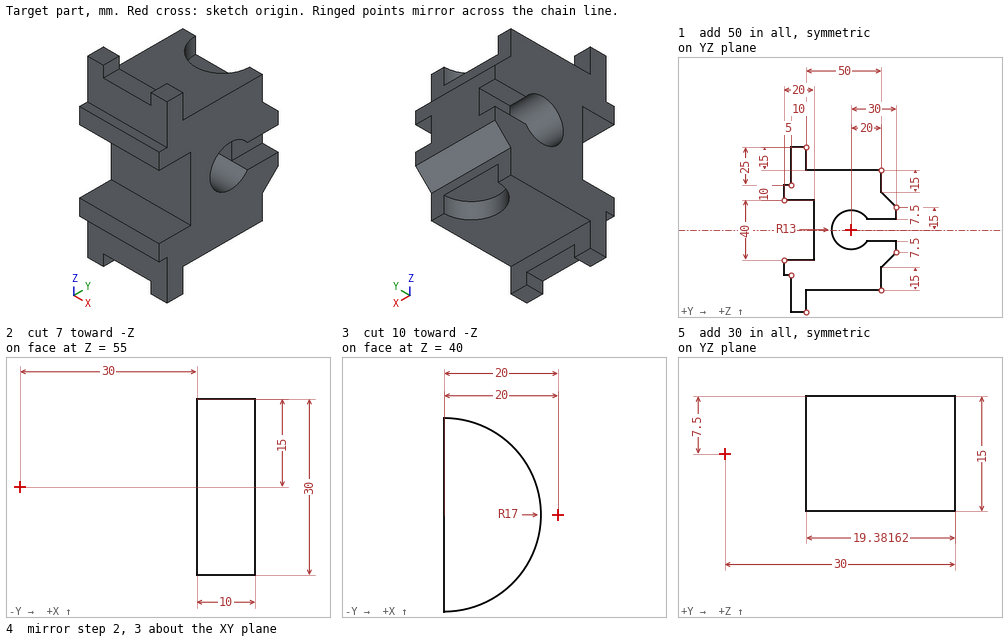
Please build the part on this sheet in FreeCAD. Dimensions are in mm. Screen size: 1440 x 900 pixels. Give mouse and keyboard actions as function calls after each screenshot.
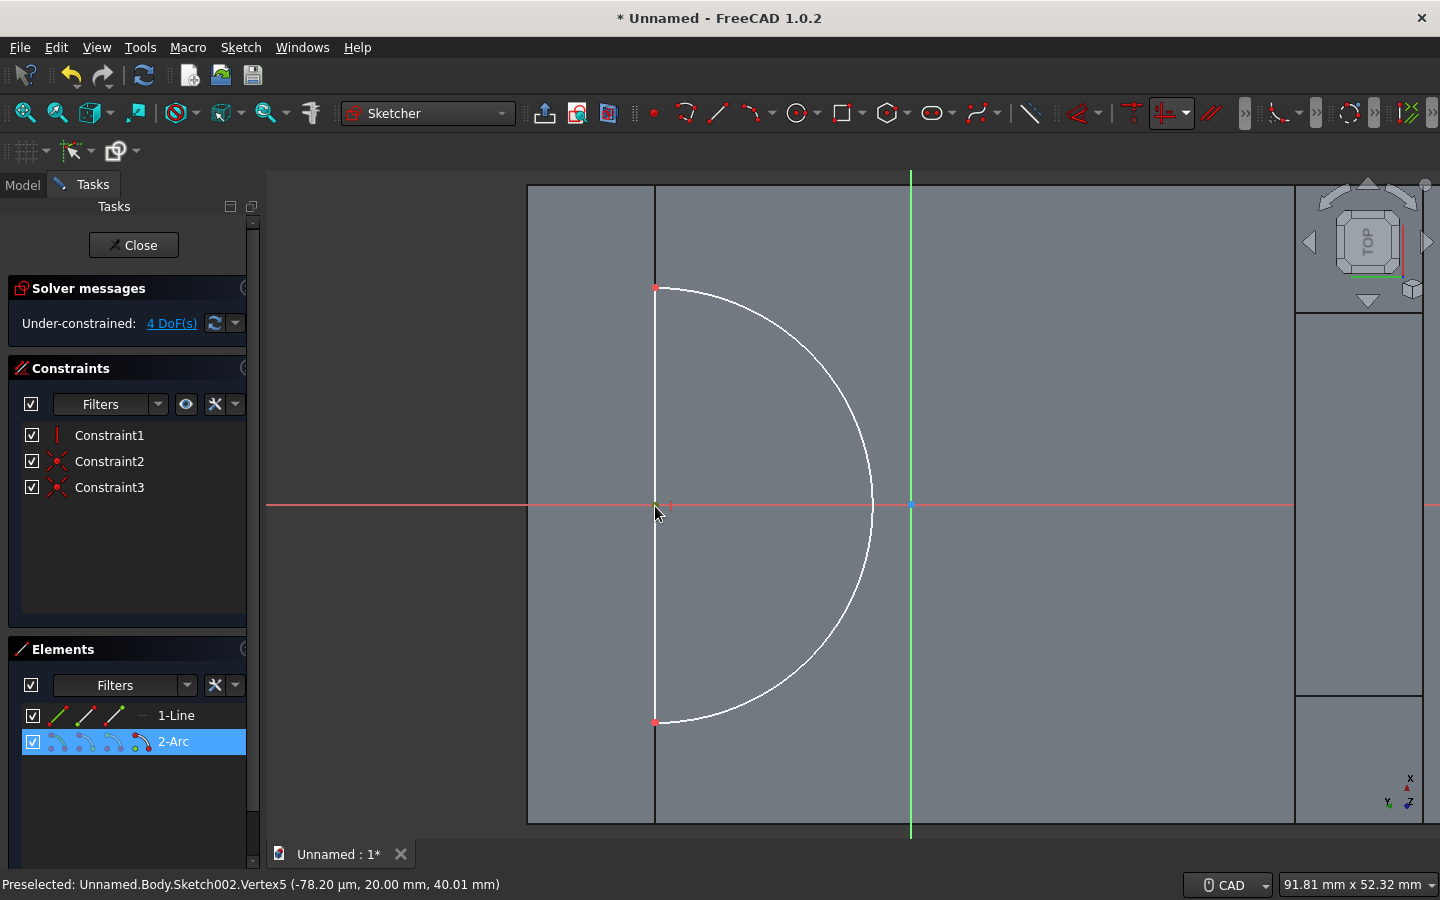
click(364, 504)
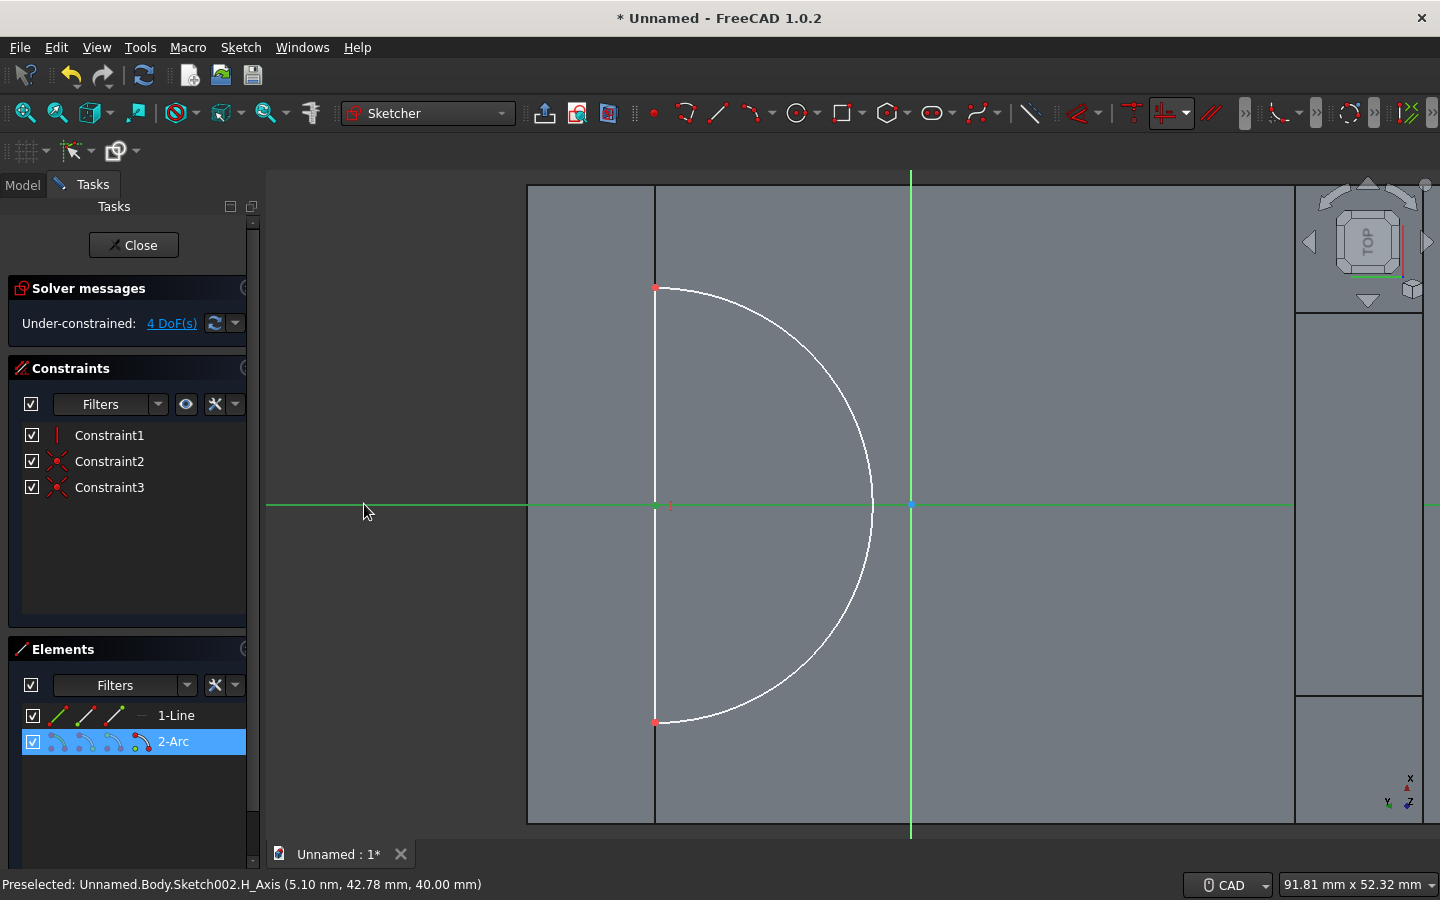
click(1132, 114)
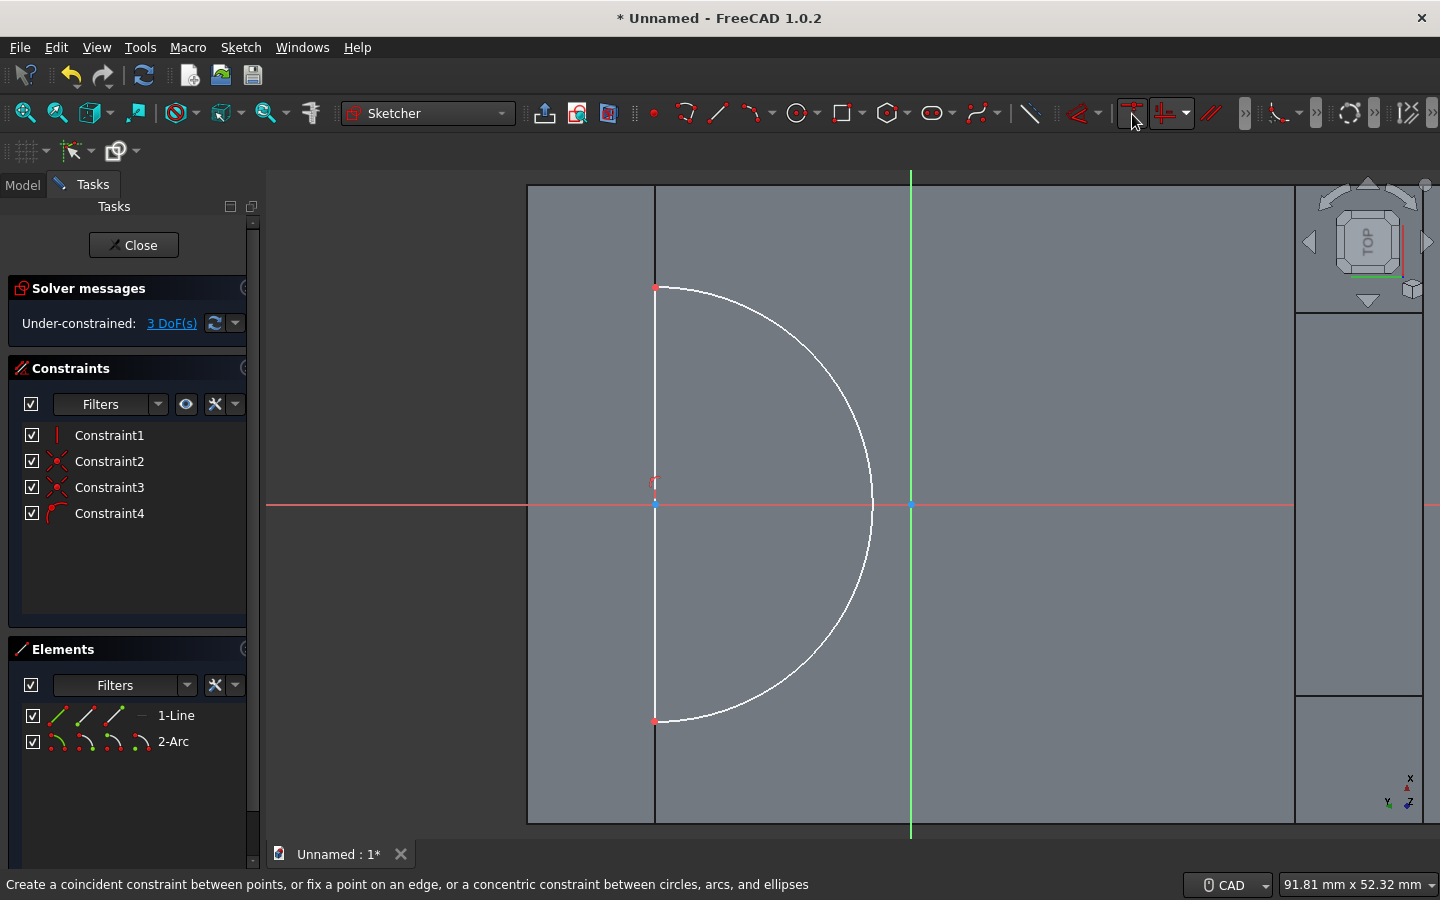
click(1078, 114)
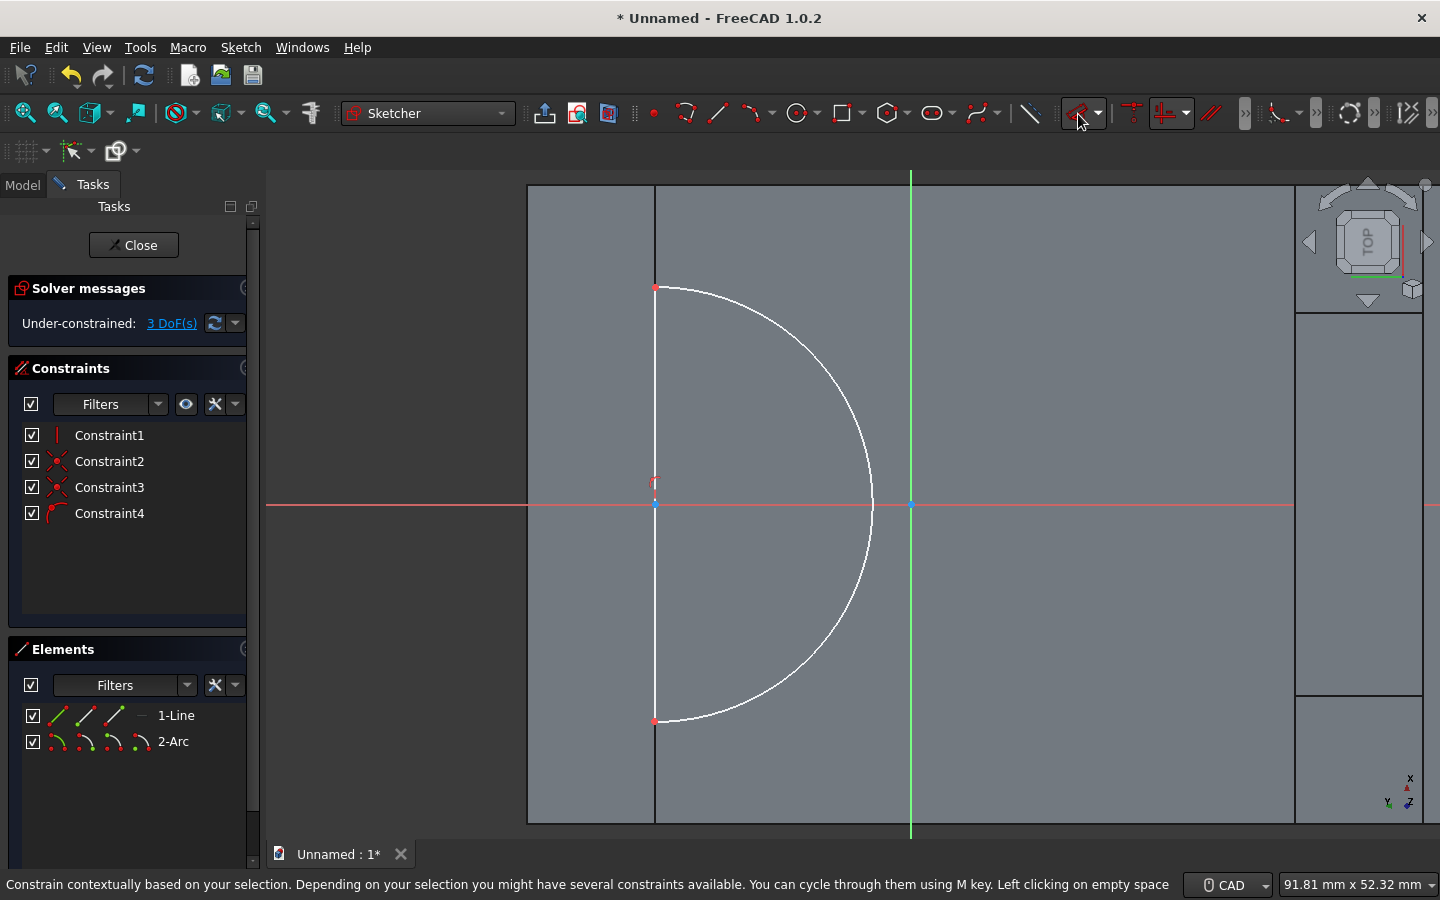
click(831, 632)
click(857, 651)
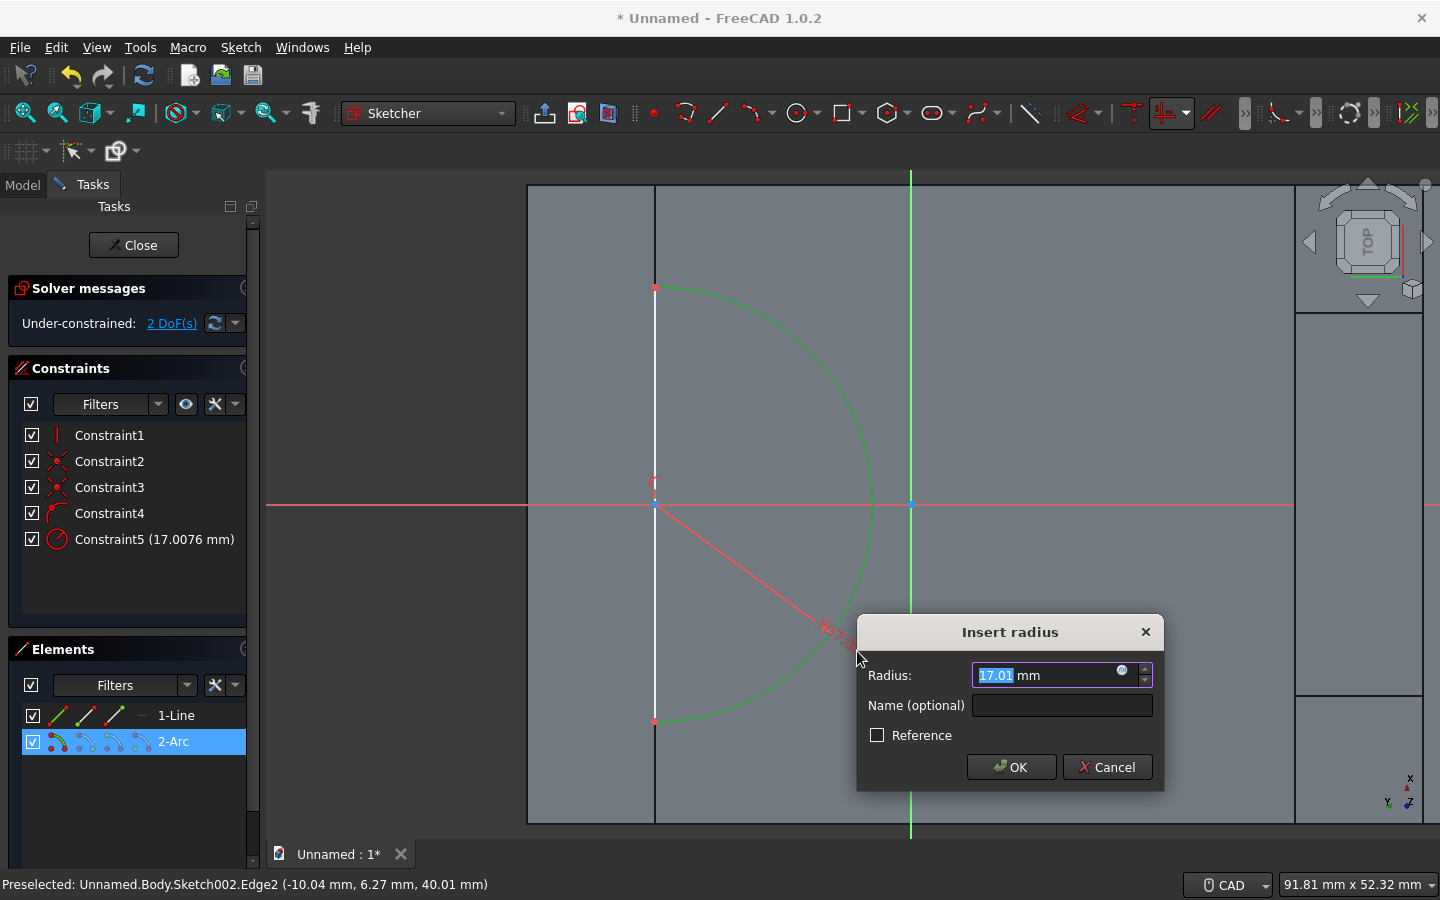
text(17)
key(Return)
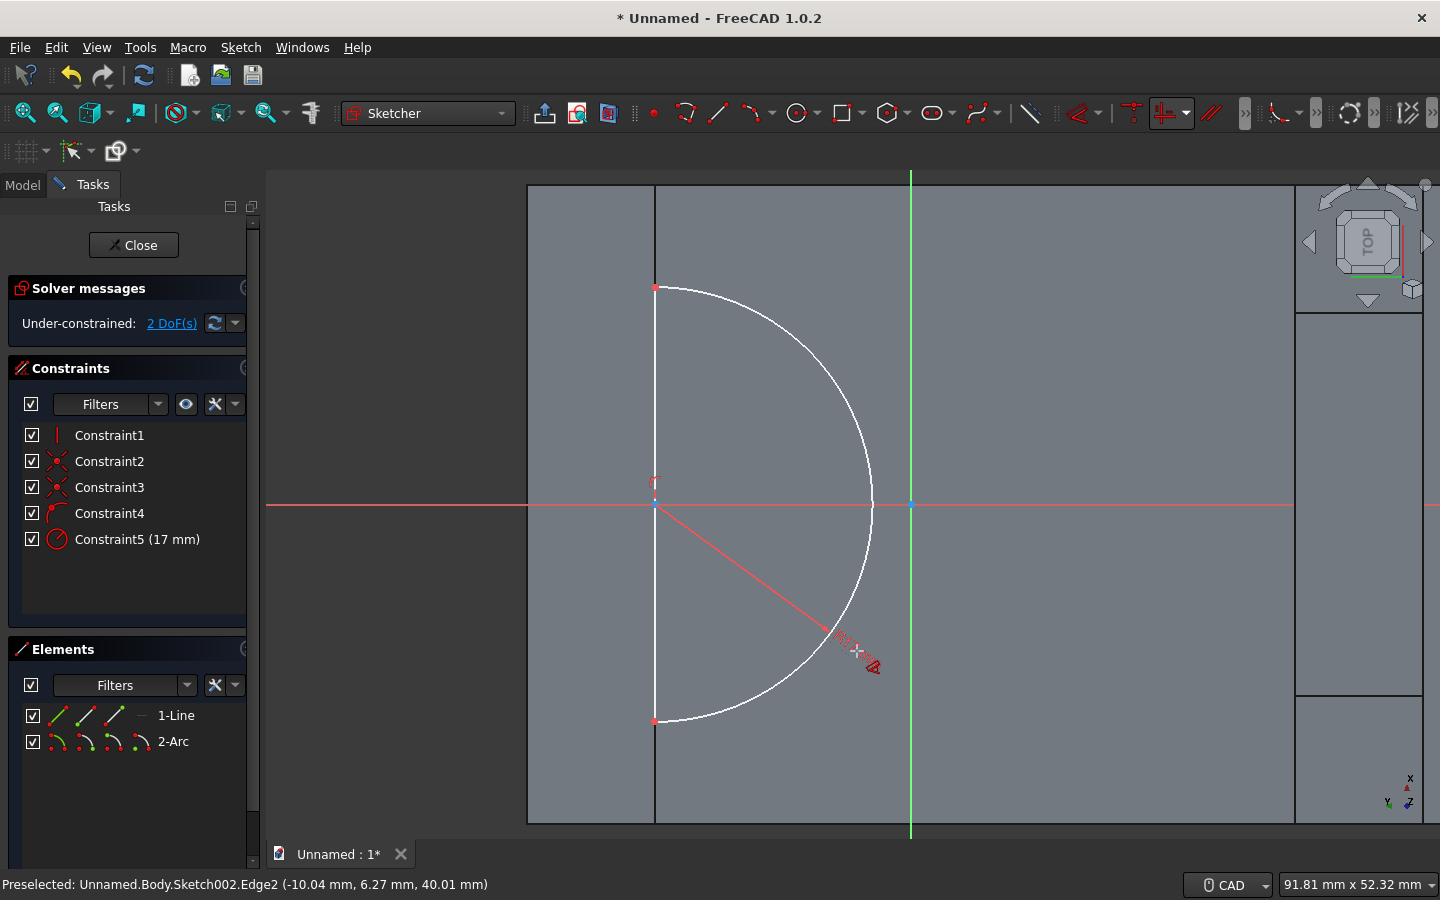
click(655, 287)
click(783, 253)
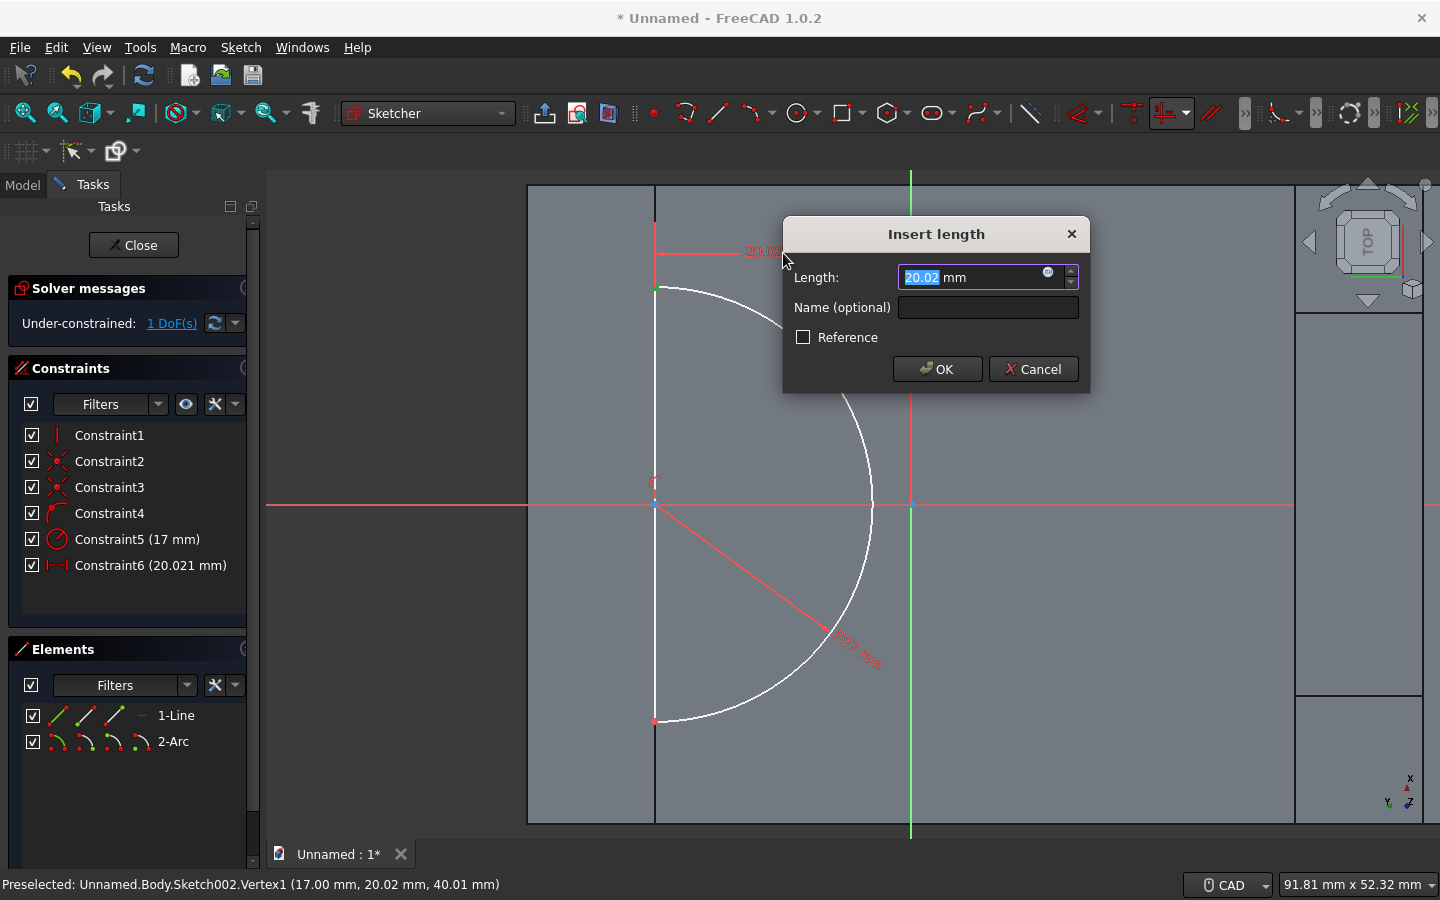
text(20)
key(Return)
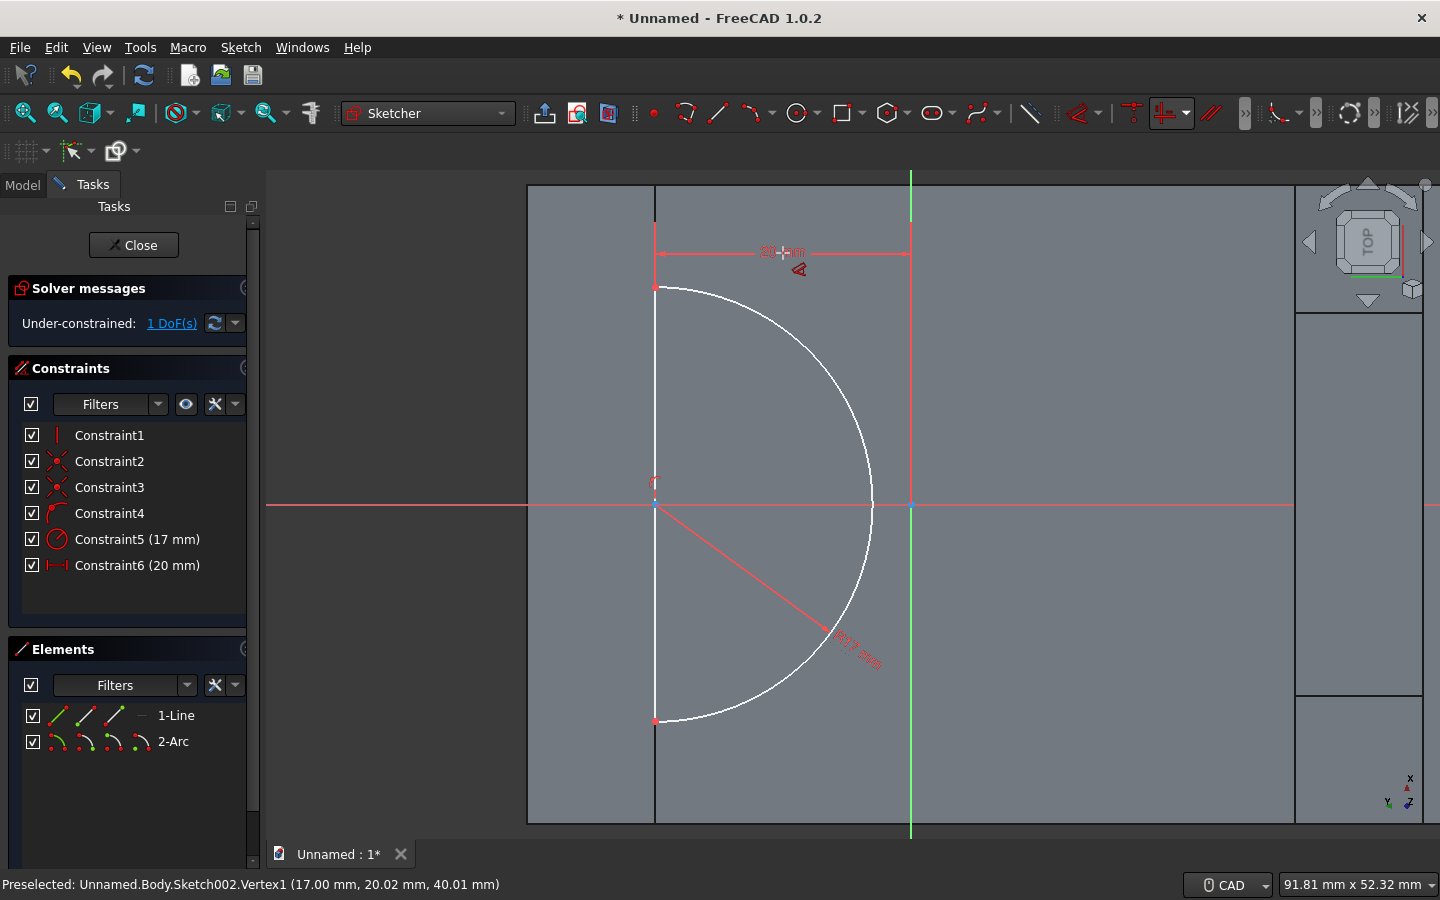
click(655, 504)
click(783, 538)